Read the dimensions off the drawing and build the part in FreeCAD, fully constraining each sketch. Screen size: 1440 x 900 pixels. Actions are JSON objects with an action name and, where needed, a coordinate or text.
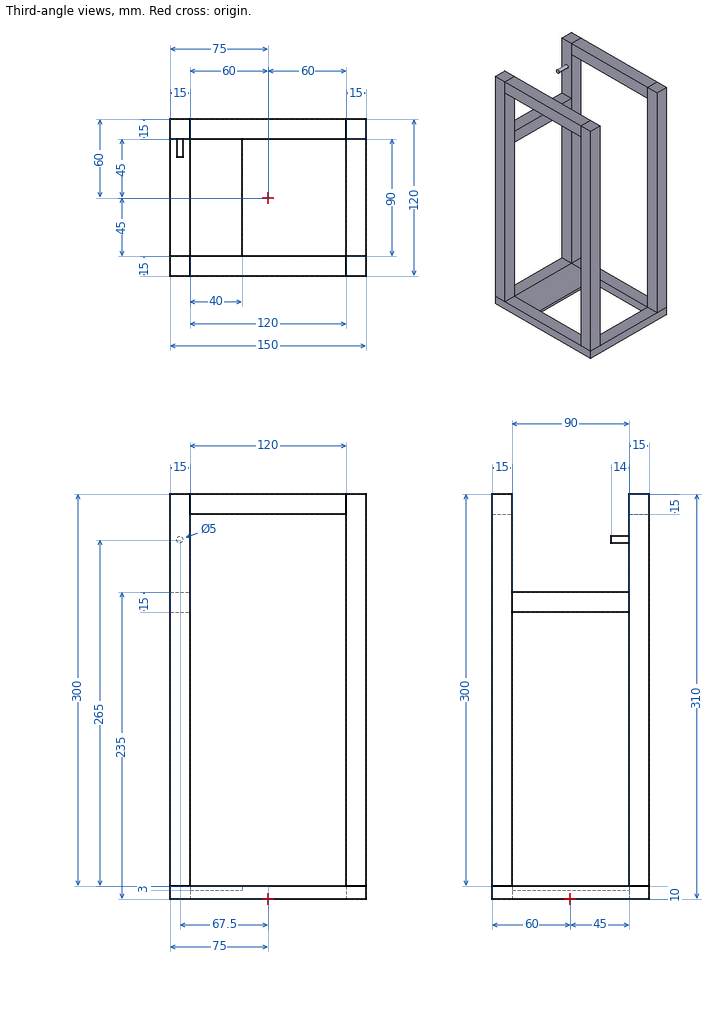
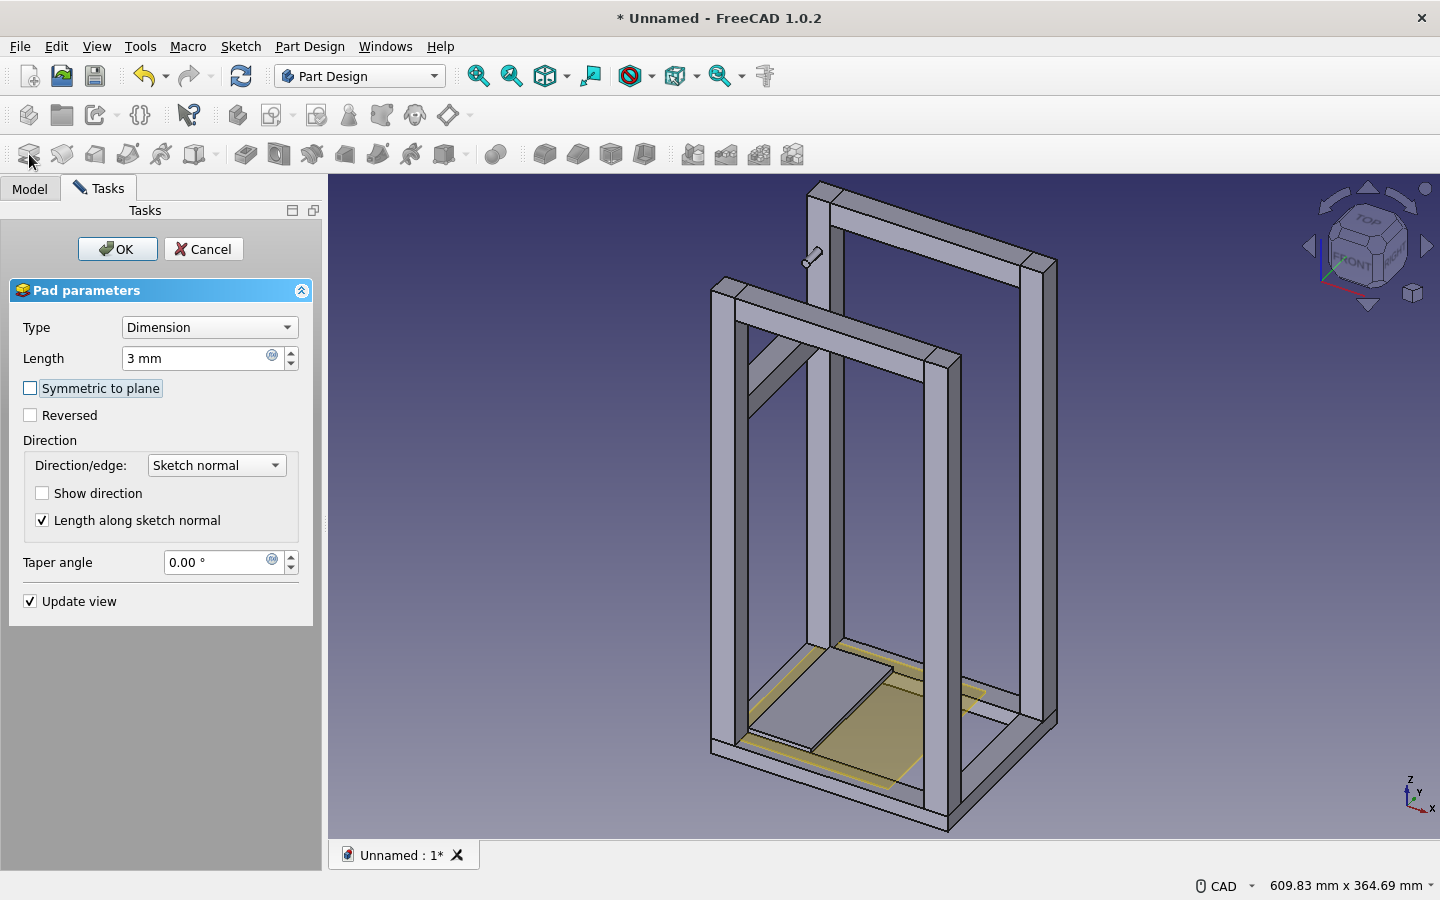
{"action": "left_click", "coordinate": [31, 415]}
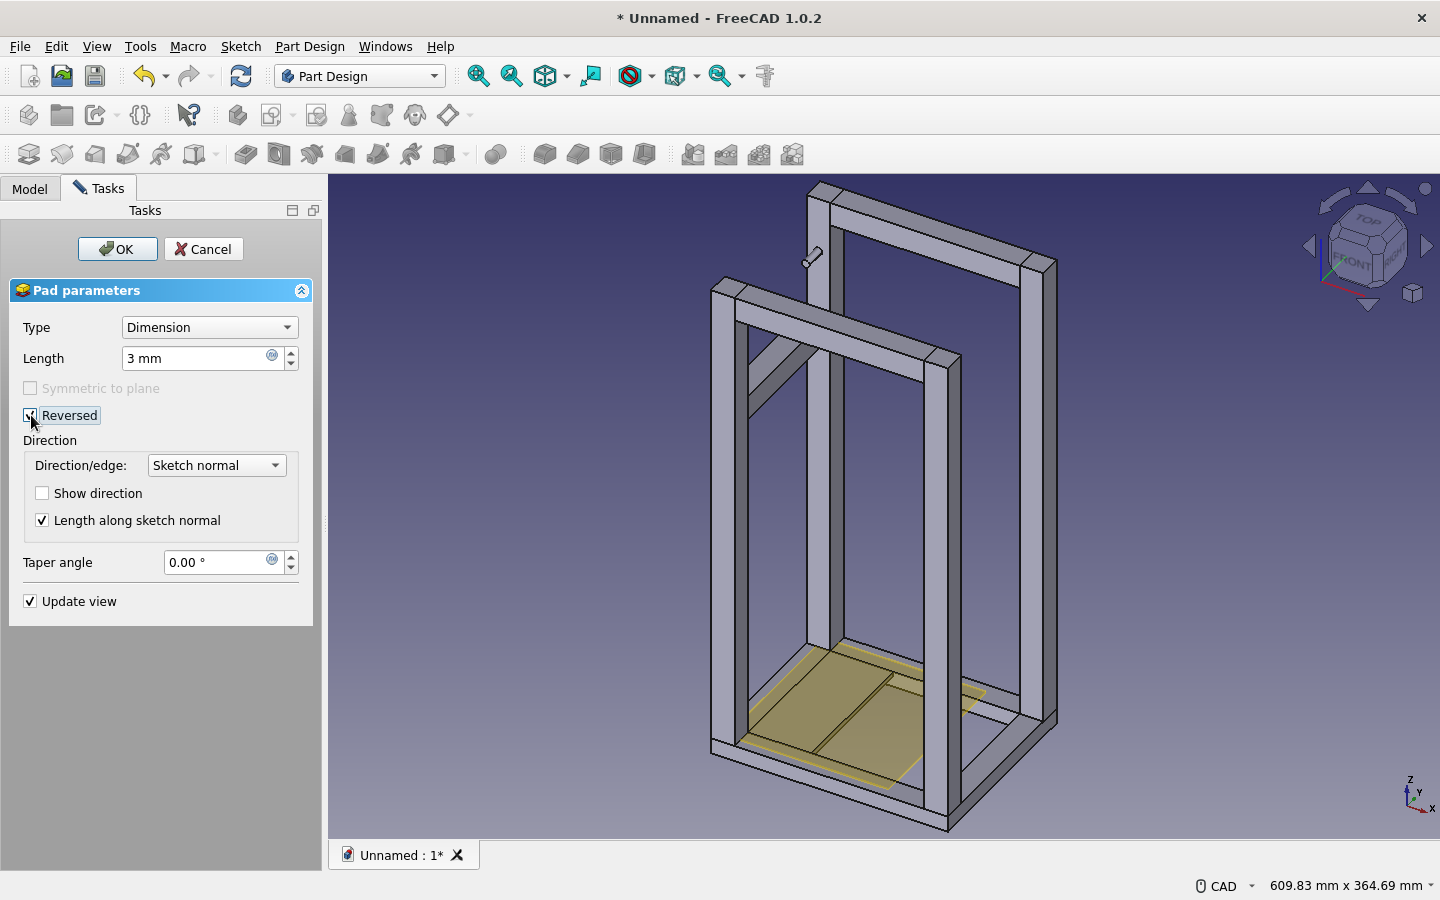
{"action": "left_click", "coordinate": [118, 249]}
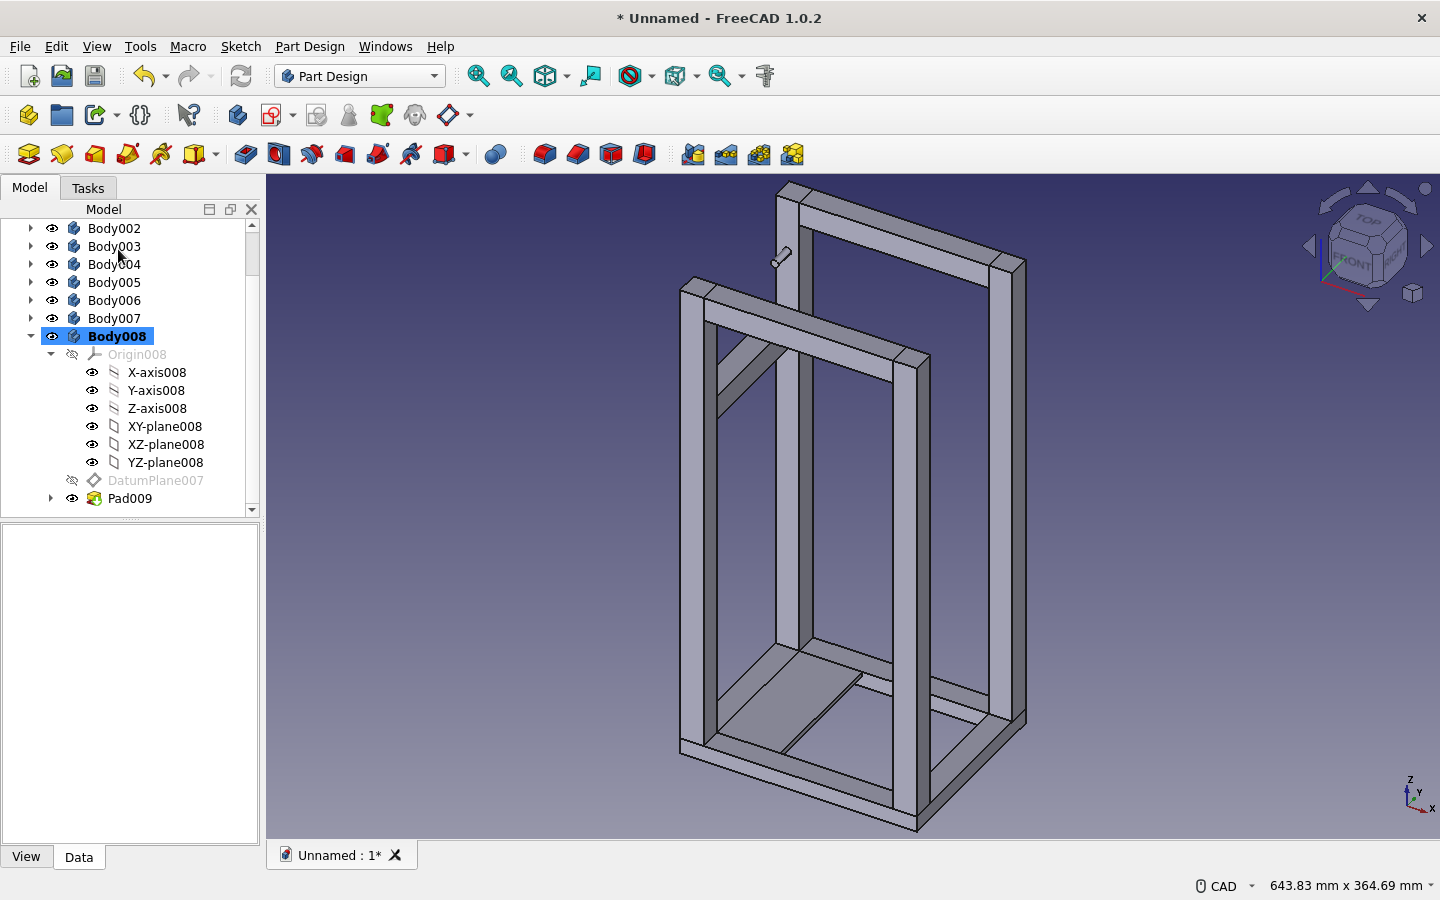
{"action": "key", "text": "0"}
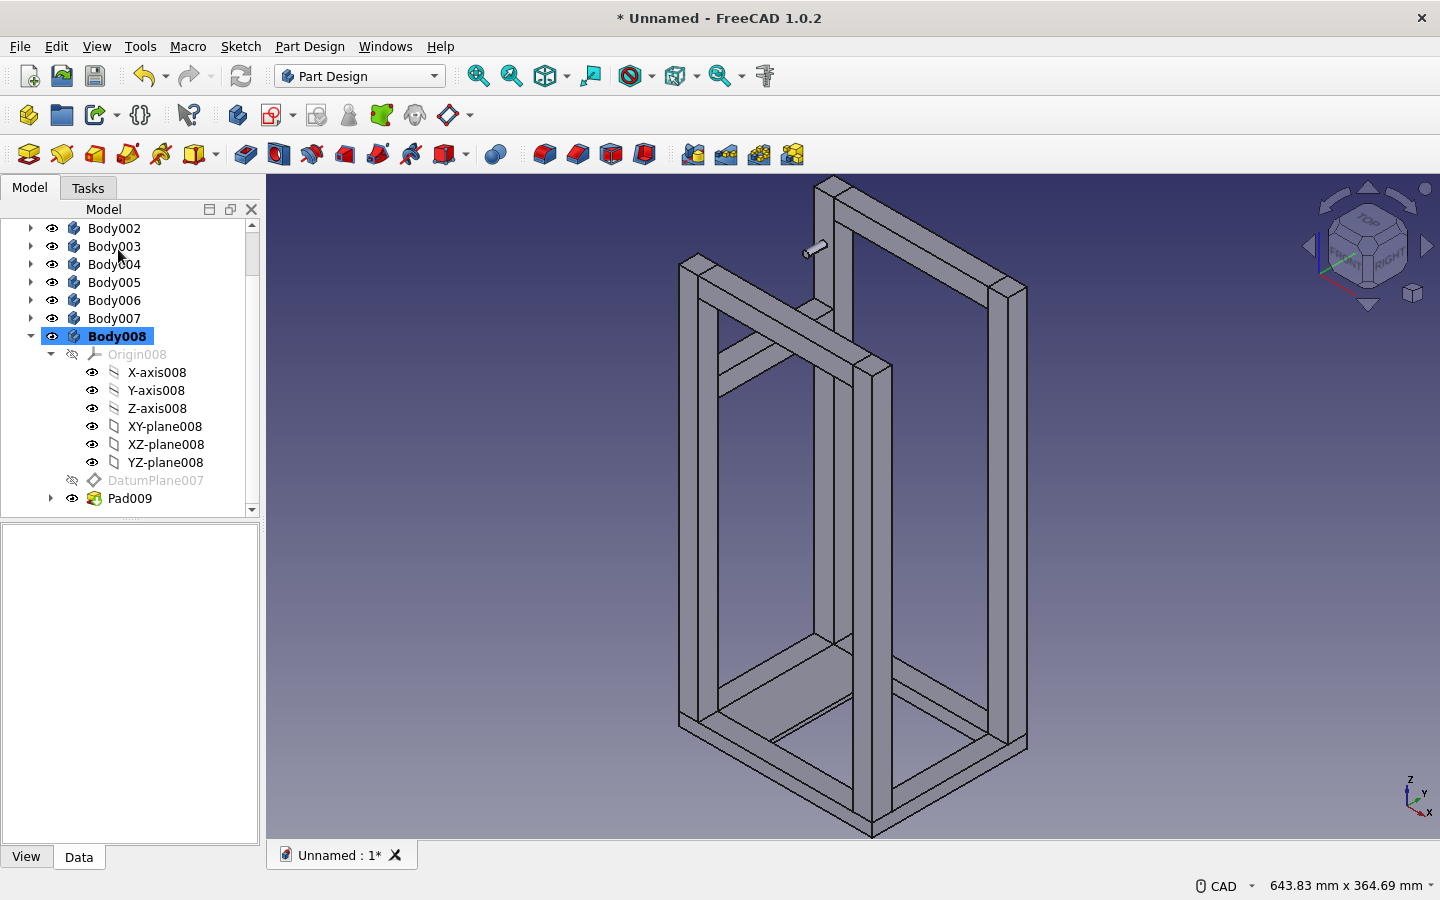
{"action": "left_click", "coordinate": [479, 76]}